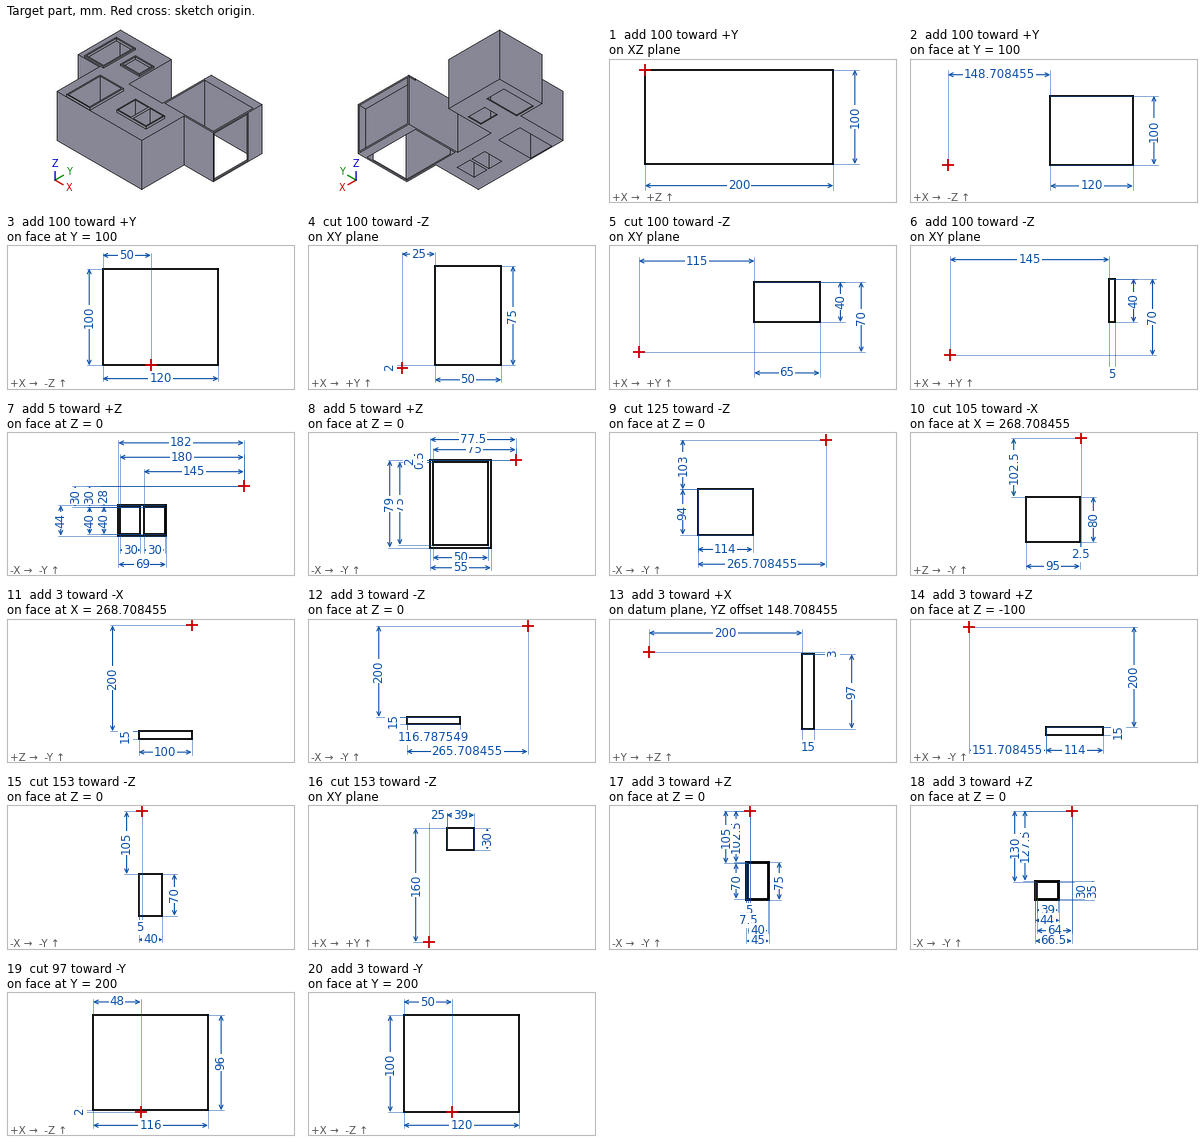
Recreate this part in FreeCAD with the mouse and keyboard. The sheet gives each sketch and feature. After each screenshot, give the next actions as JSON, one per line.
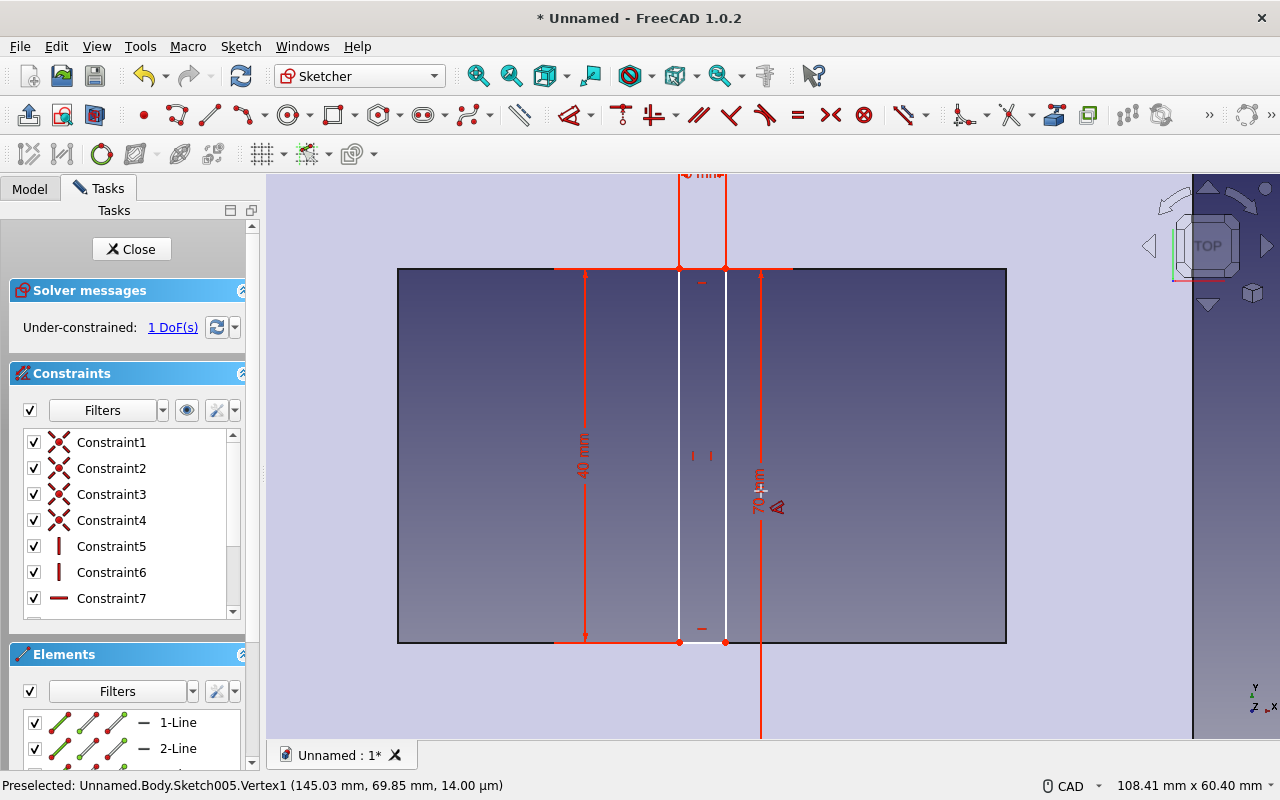
{"action": "left_click", "coordinate": [679, 269]}
{"action": "left_click", "coordinate": [486, 235]}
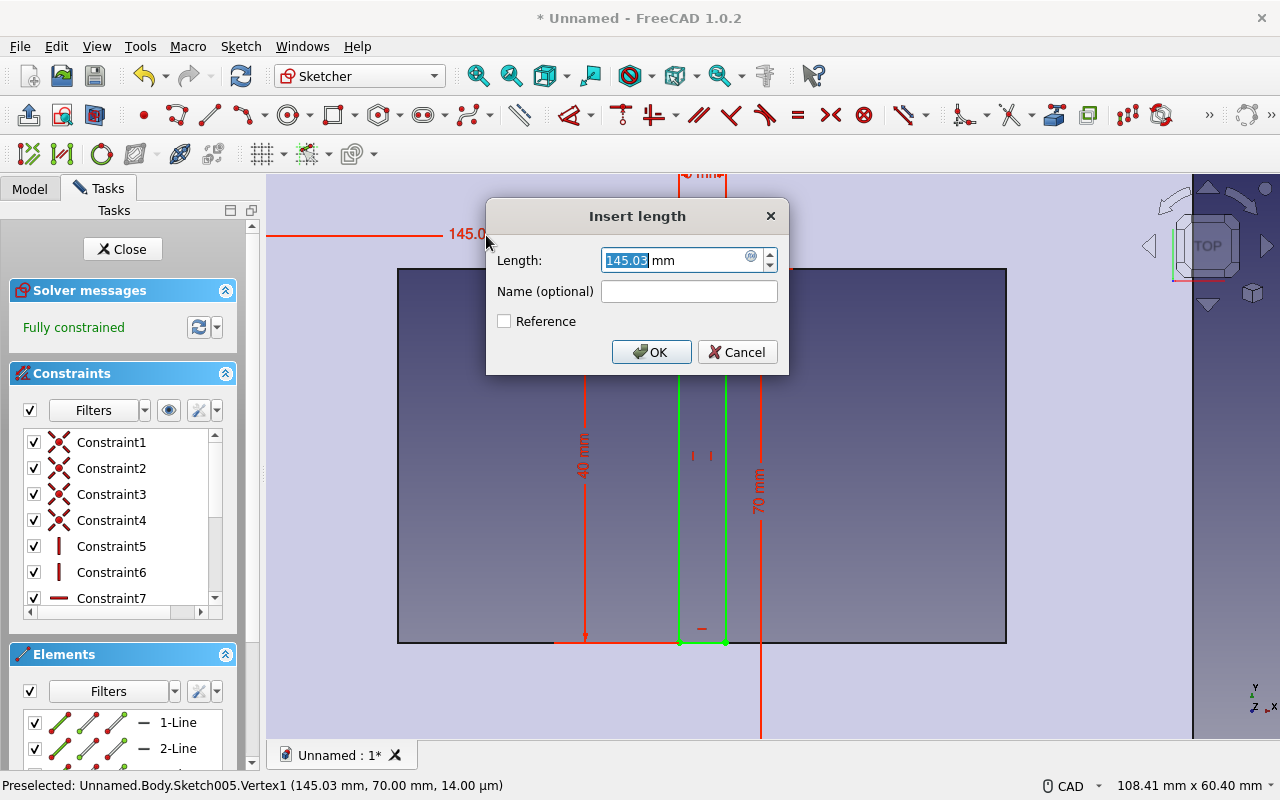
{"action": "type", "text": "145"}
{"action": "key", "text": "Return"}
{"action": "key", "text": "Escape"}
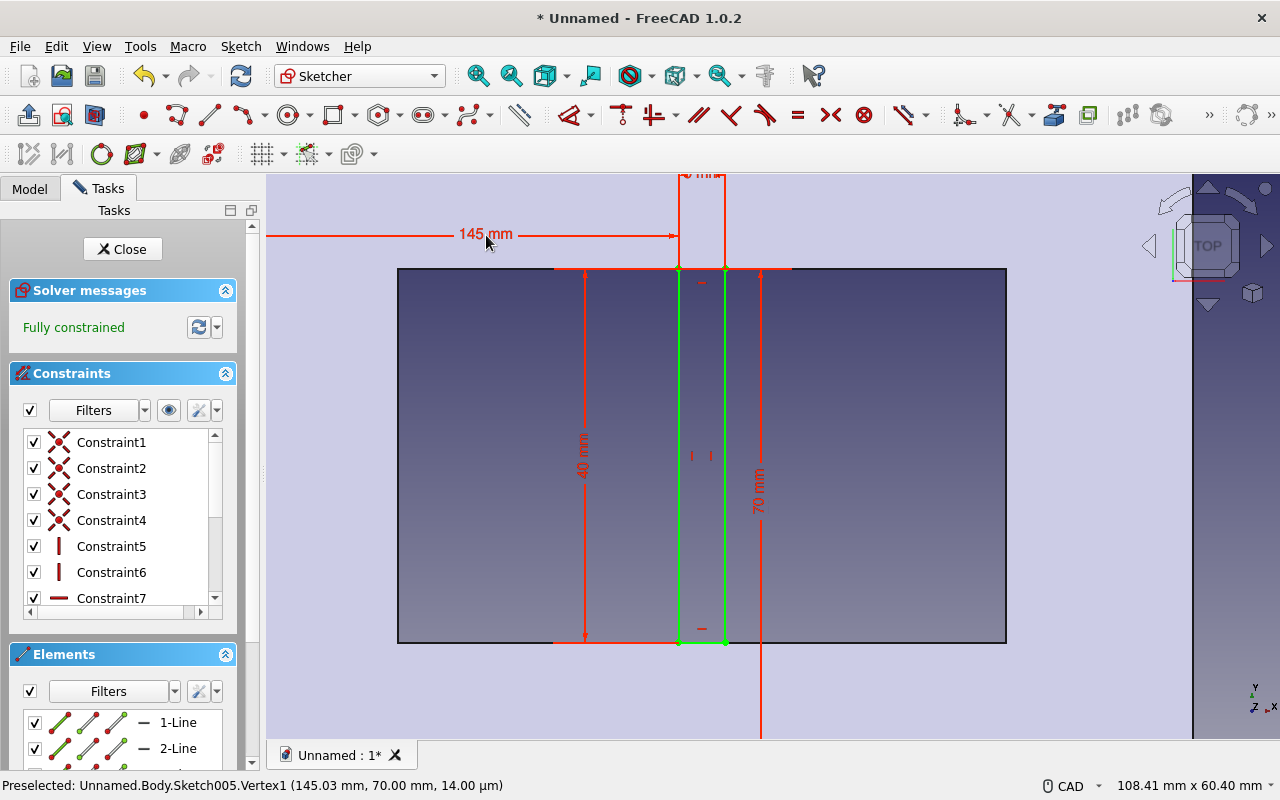
{"action": "left_click", "coordinate": [123, 249]}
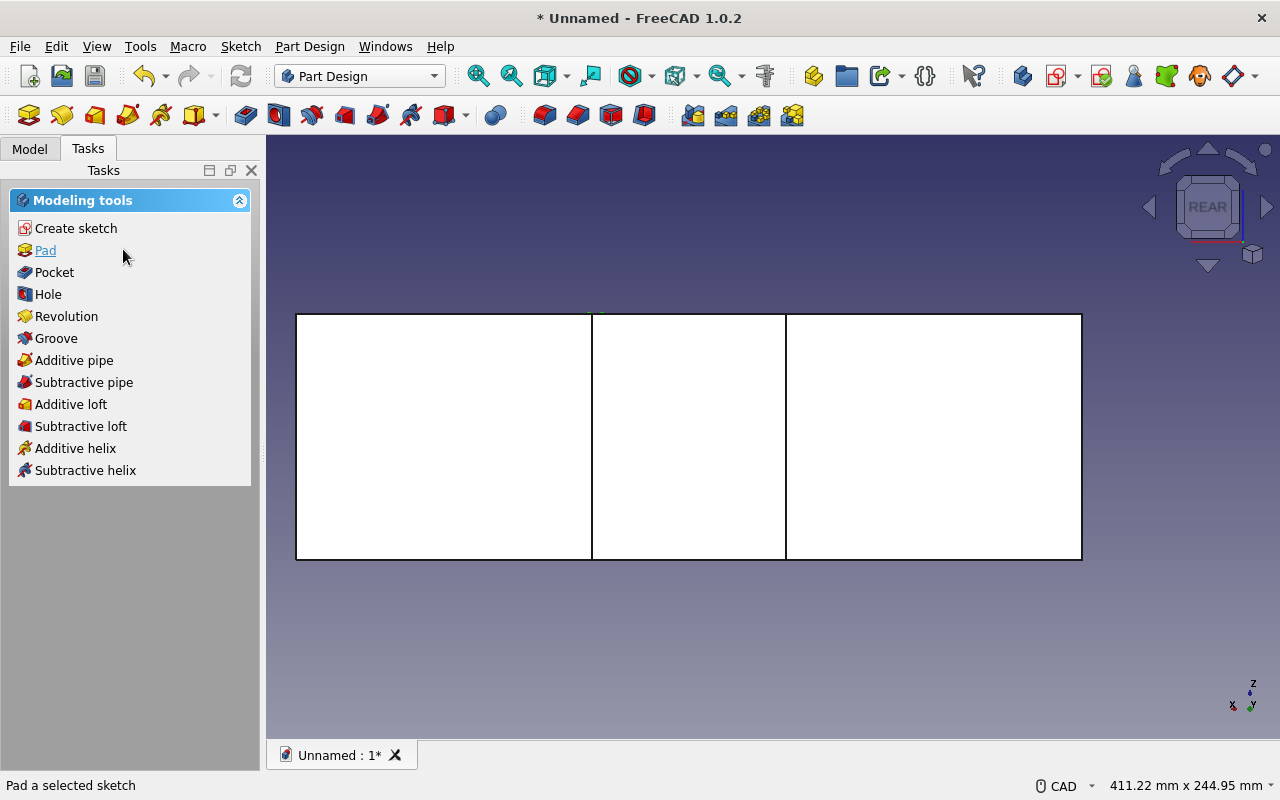
{"action": "left_click", "coordinate": [29, 116]}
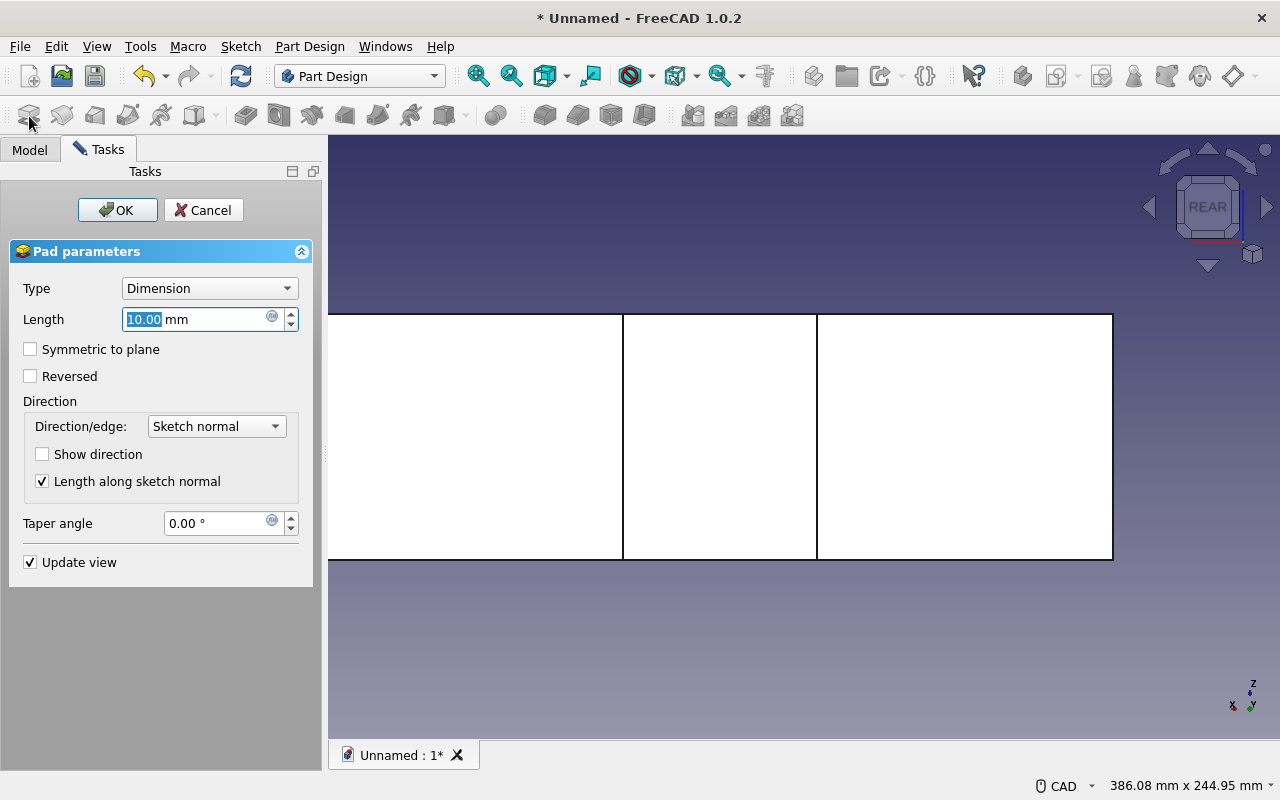
{"action": "type", "text": "100"}
{"action": "key", "text": "Tab"}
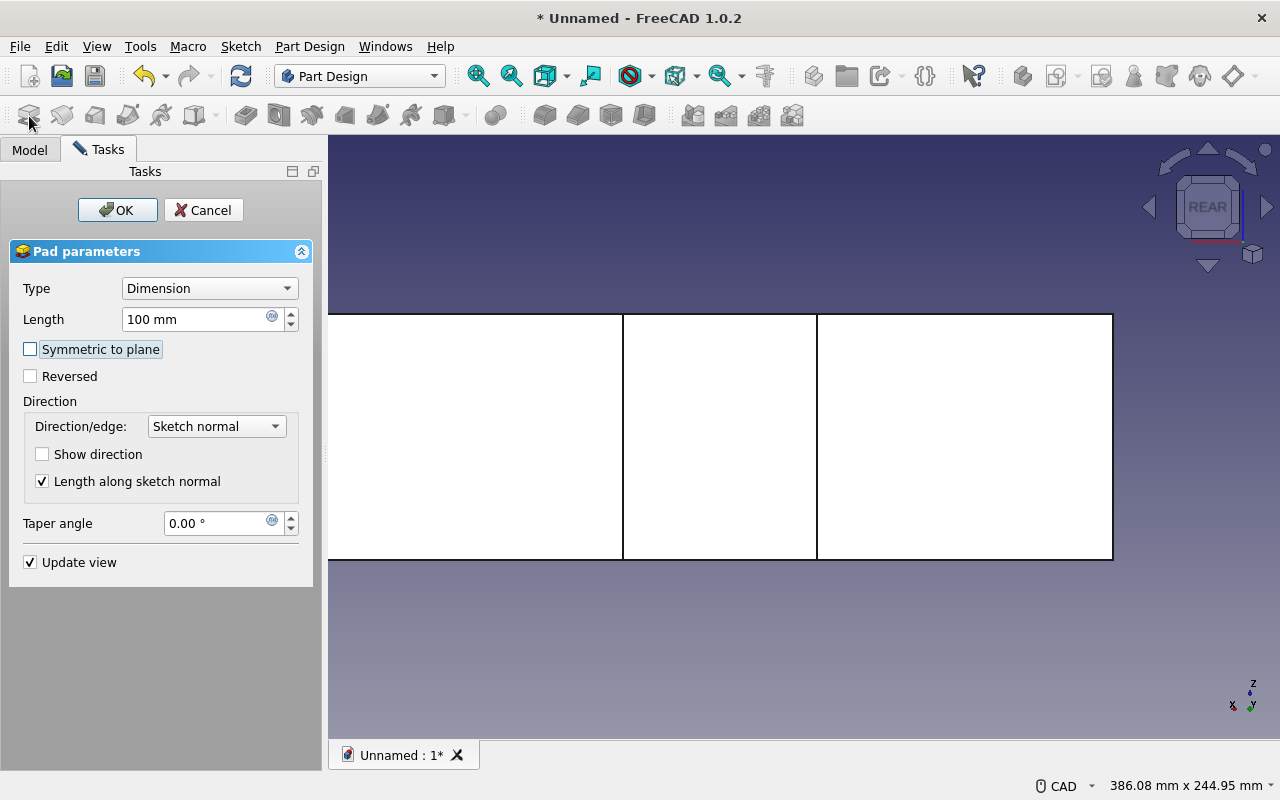
{"action": "left_click", "coordinate": [31, 376]}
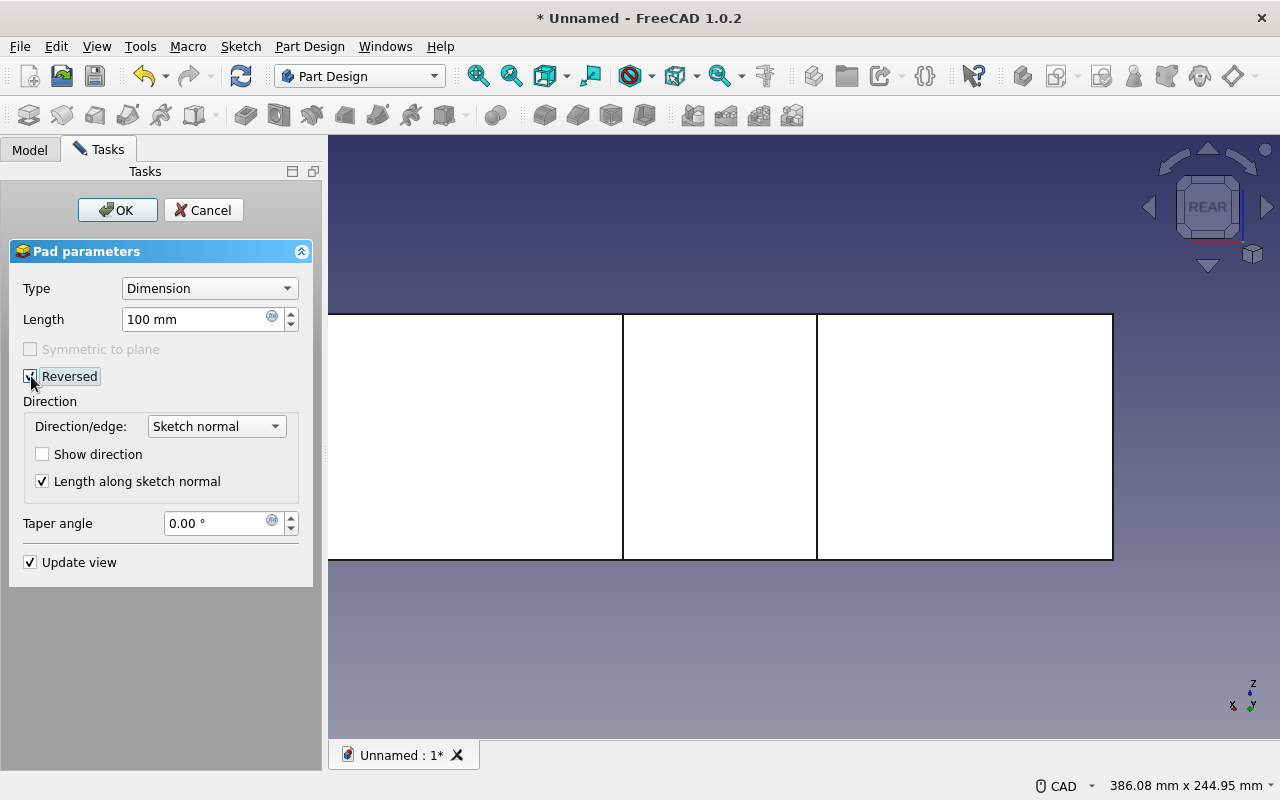
{"action": "left_click", "coordinate": [118, 210]}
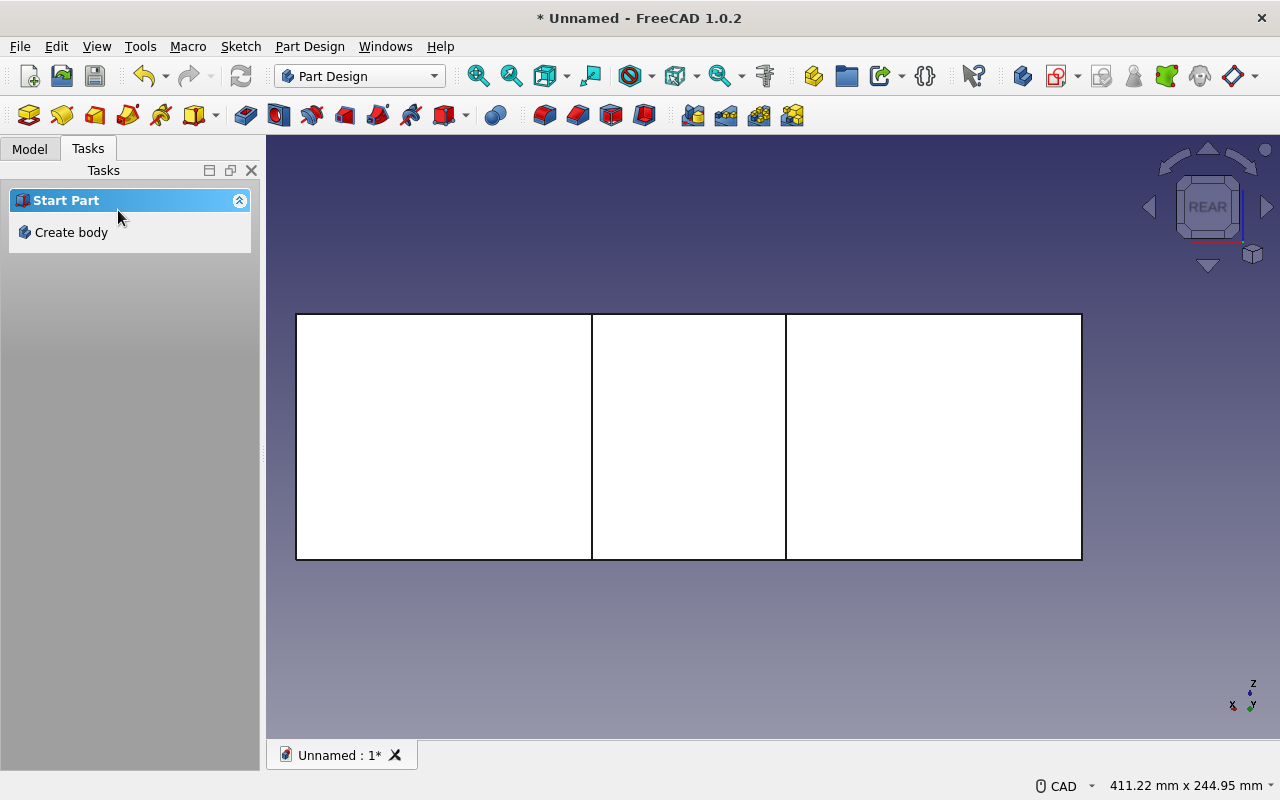
{"action": "key", "text": "0"}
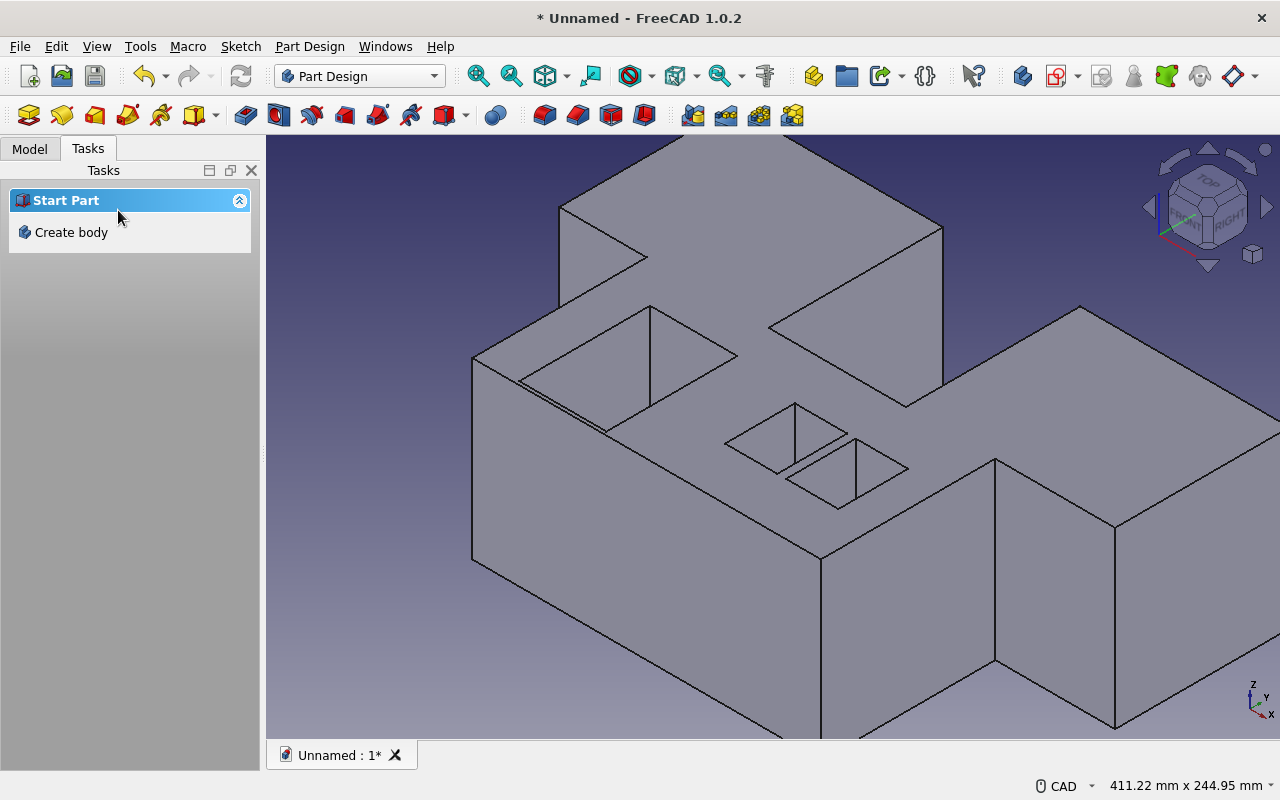
{"action": "left_click", "coordinate": [479, 76]}